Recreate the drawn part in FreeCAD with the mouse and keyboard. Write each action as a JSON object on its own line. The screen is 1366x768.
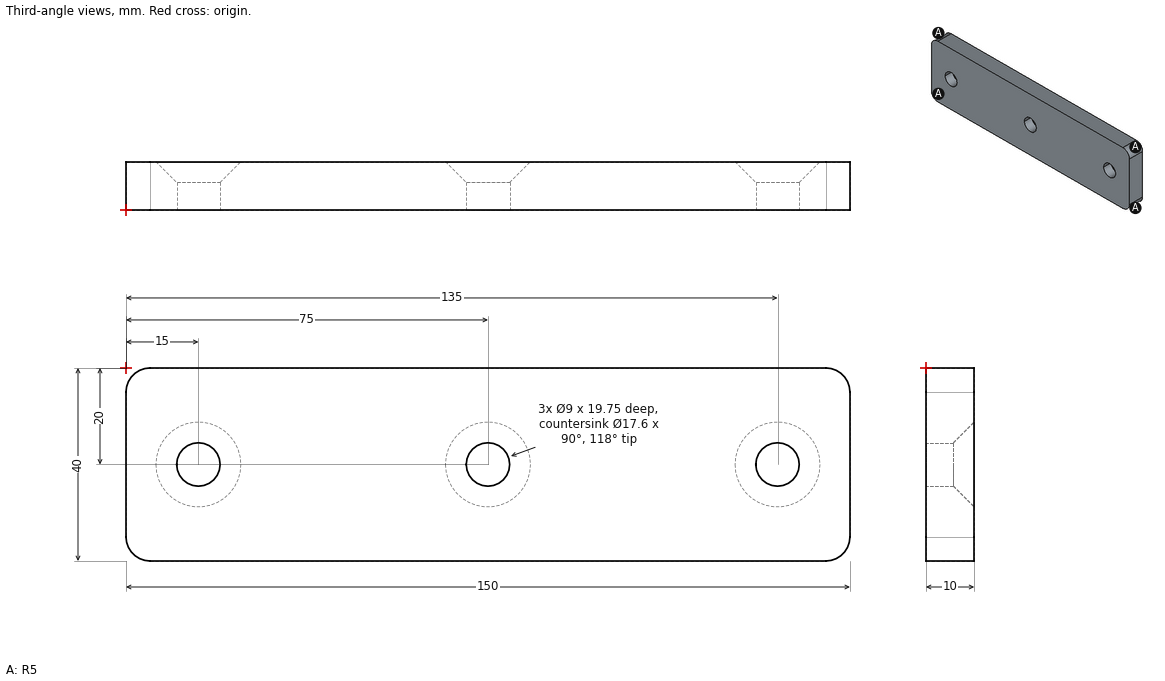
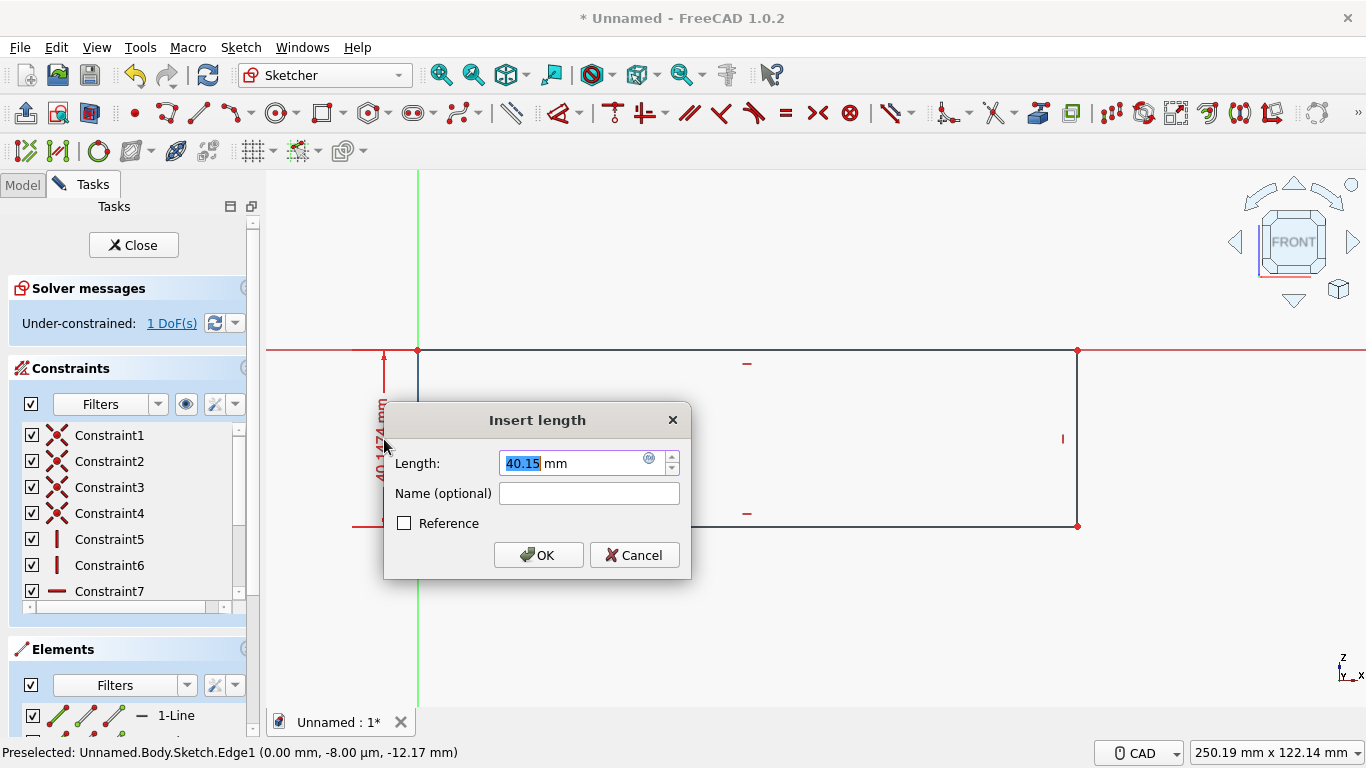
{"action": "type", "text": "40"}
{"action": "key", "text": "Return"}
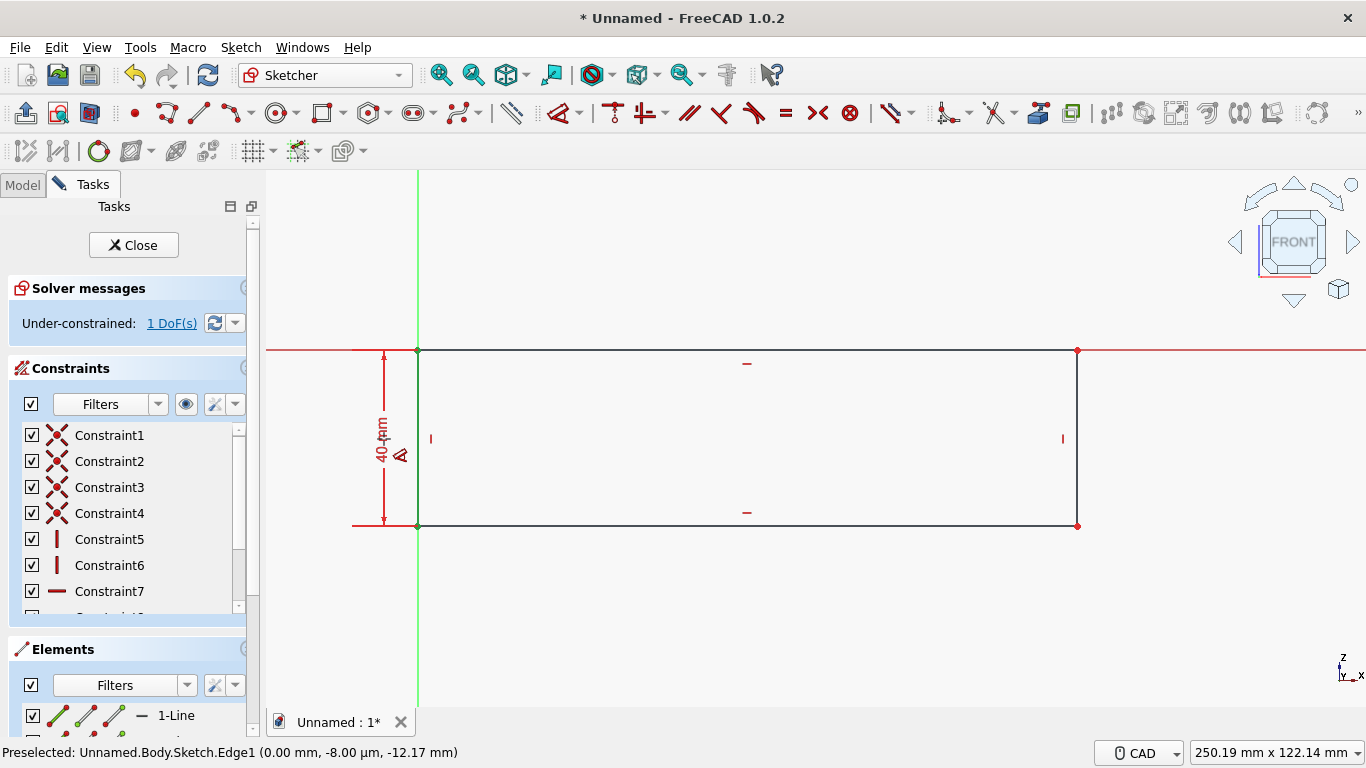
{"action": "left_click", "coordinate": [615, 526]}
{"action": "left_click", "coordinate": [747, 560]}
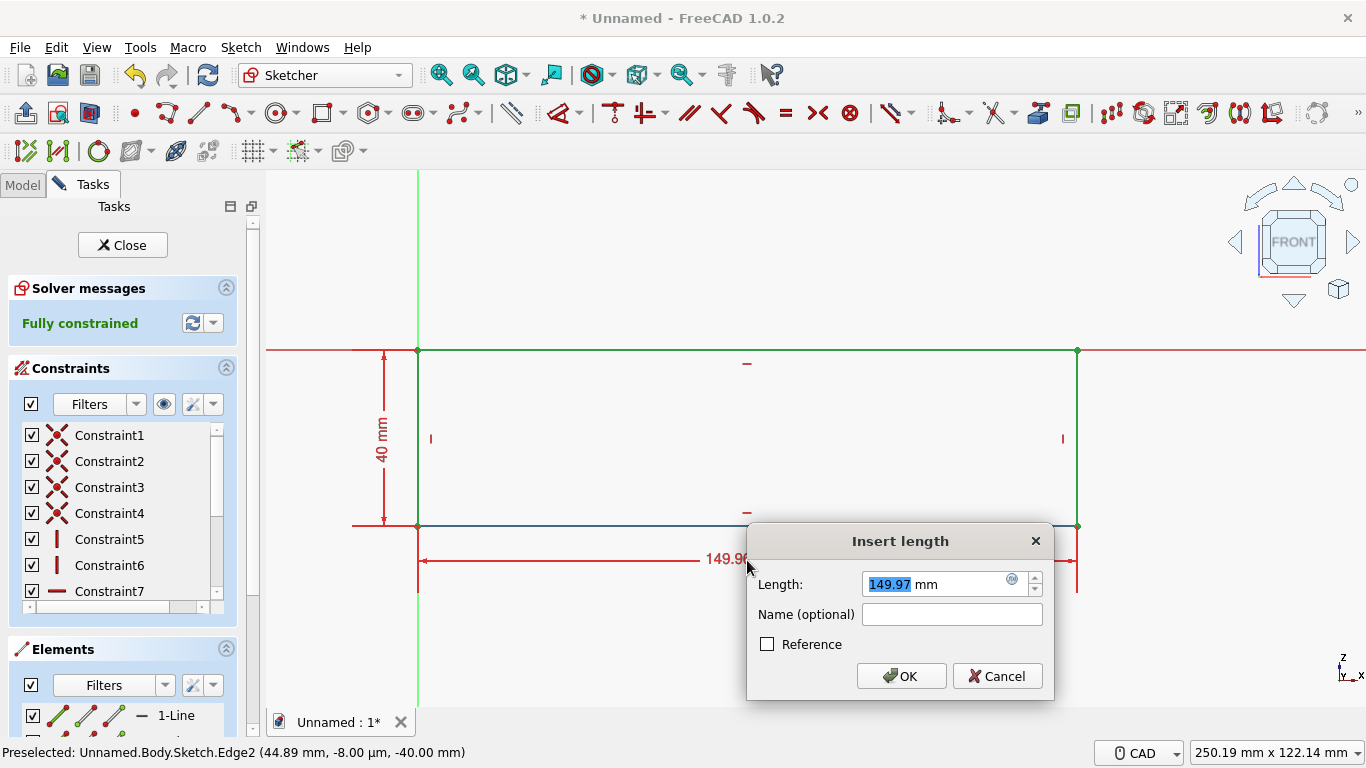
{"action": "type", "text": "150"}
{"action": "key", "text": "Return"}
{"action": "key", "text": "Escape"}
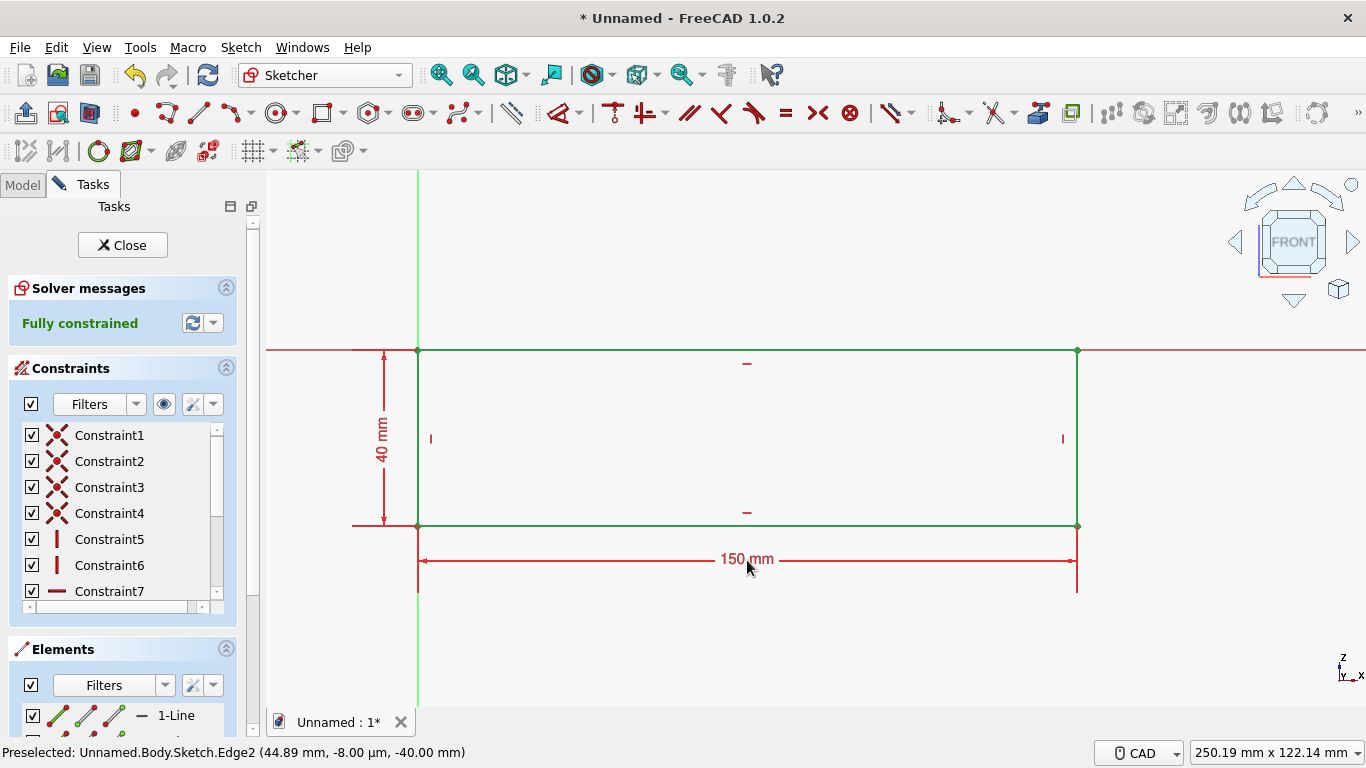
{"action": "left_click", "coordinate": [123, 245]}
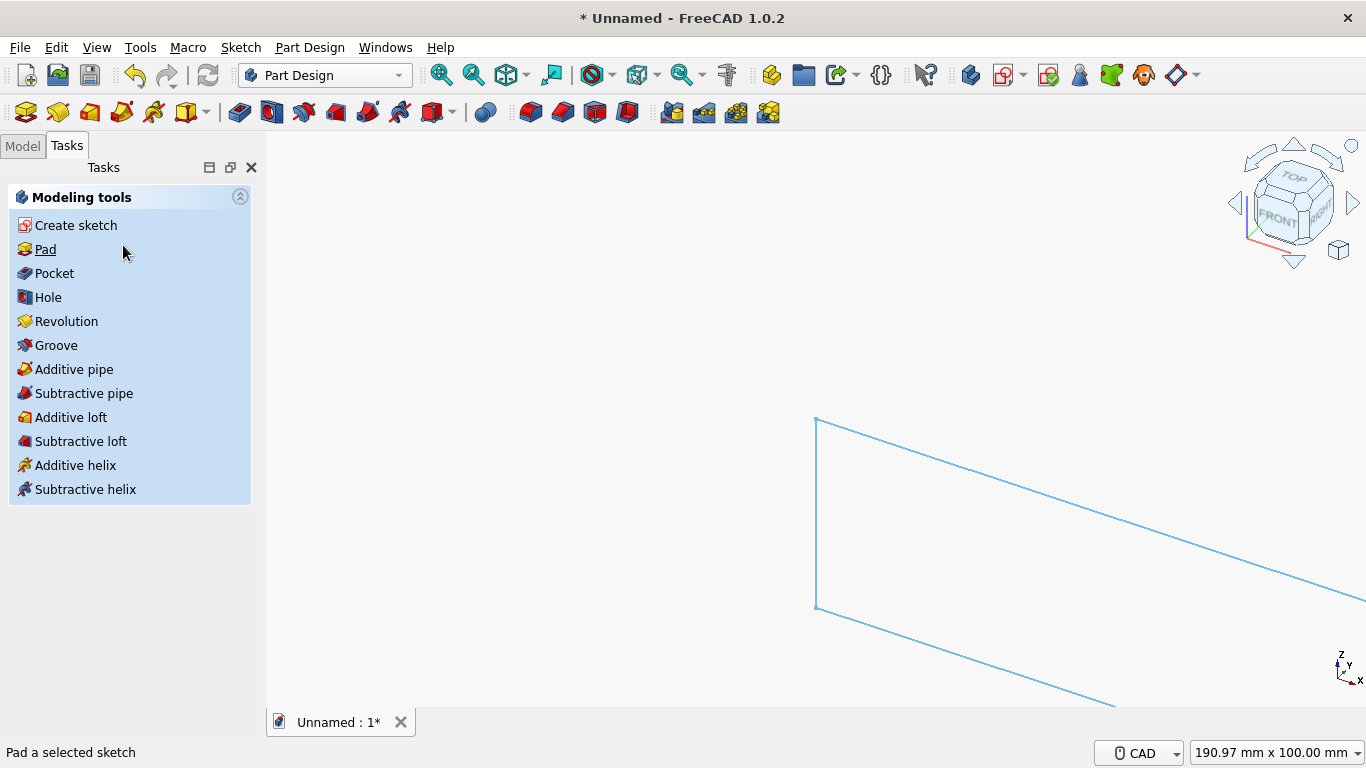
{"action": "left_click", "coordinate": [26, 112]}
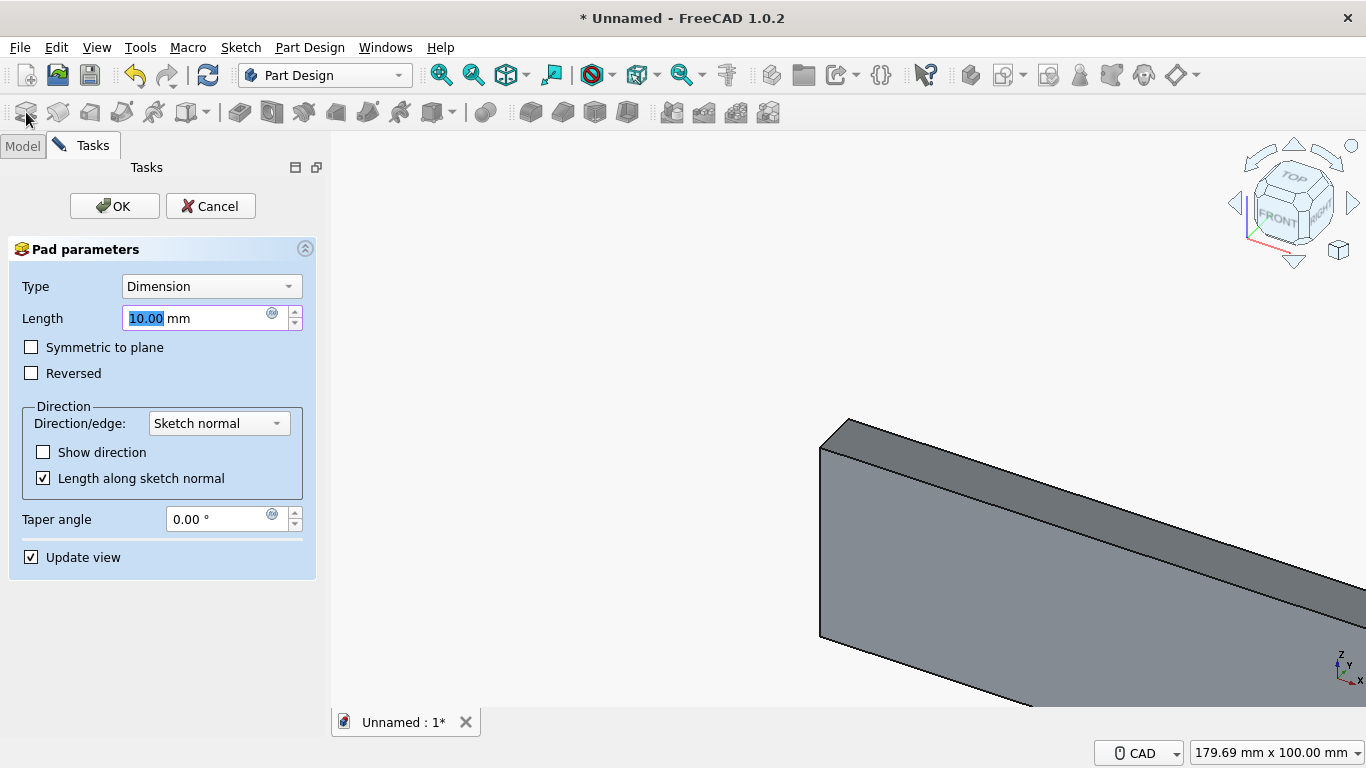
{"action": "type", "text": "10"}
{"action": "key", "text": "Tab"}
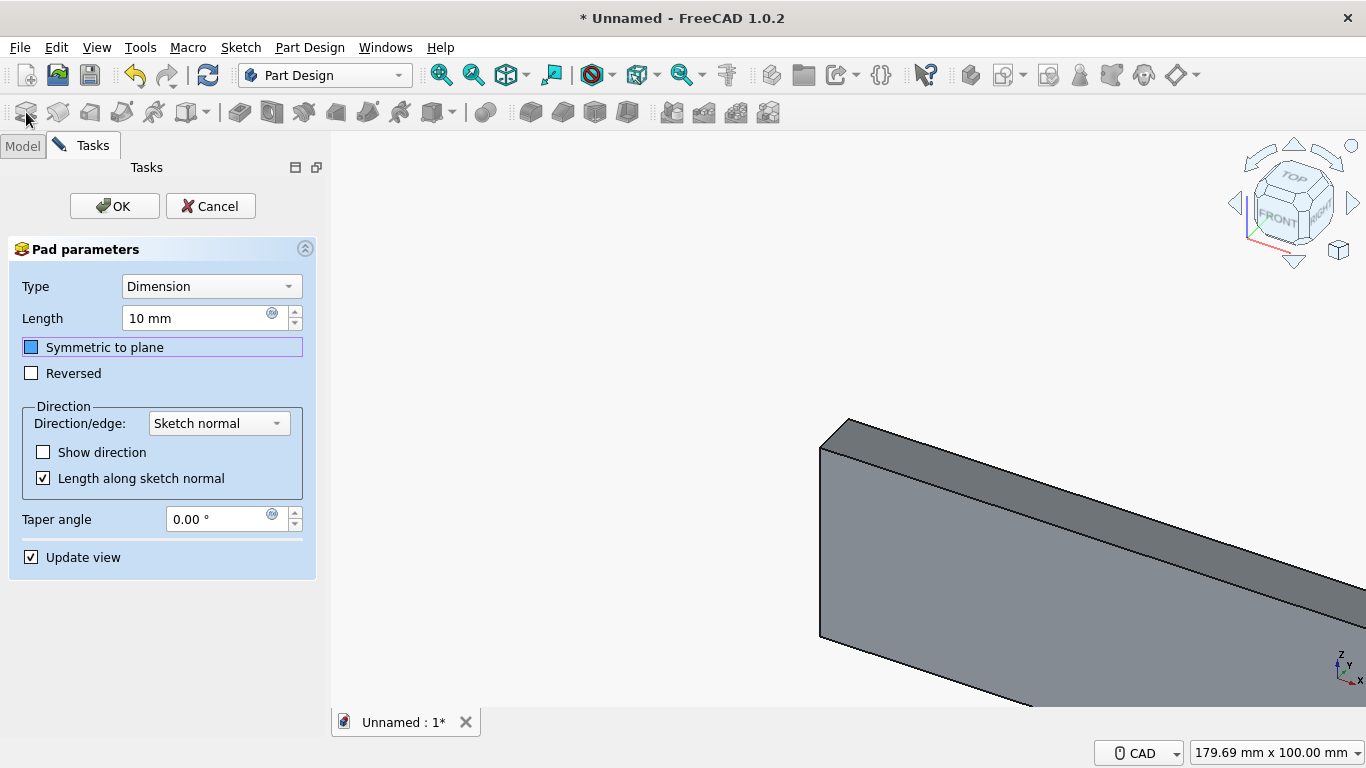
{"action": "left_click", "coordinate": [30, 373]}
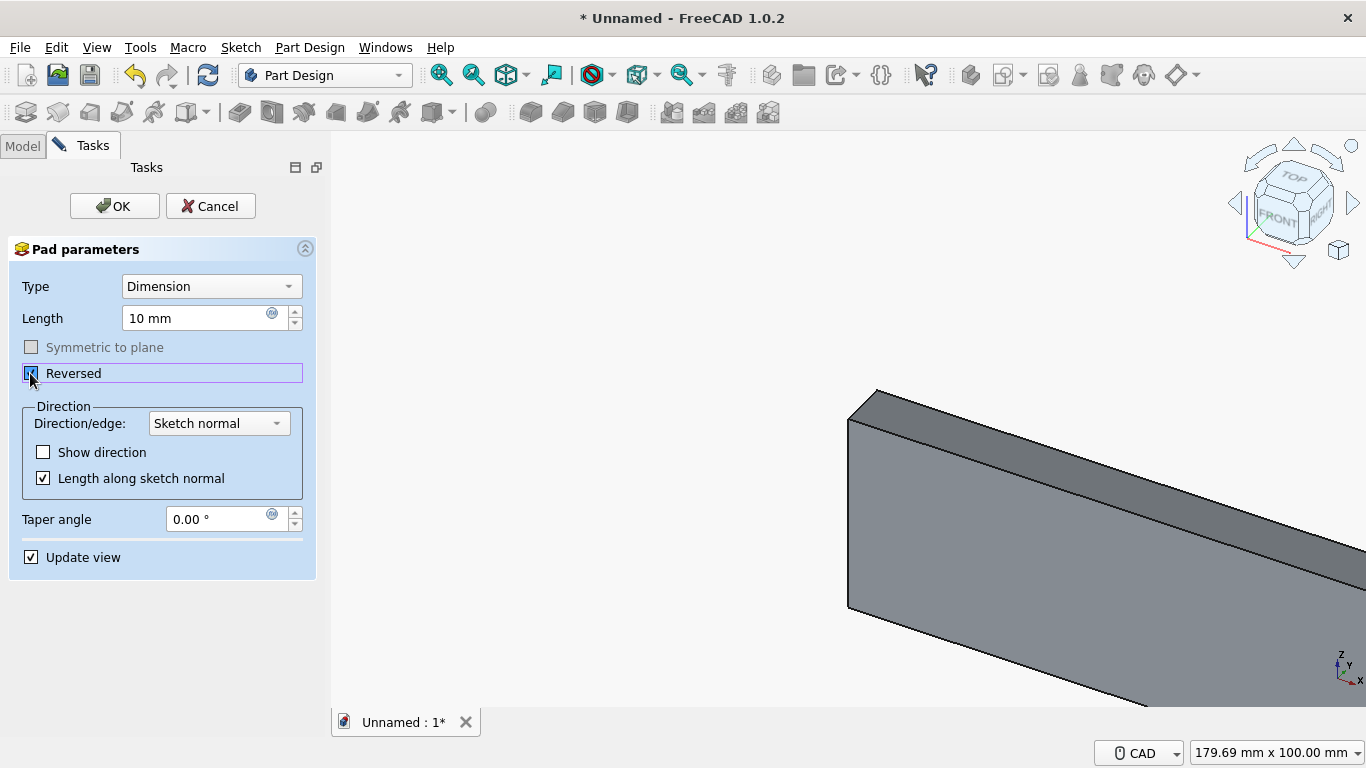
{"action": "left_click", "coordinate": [115, 206]}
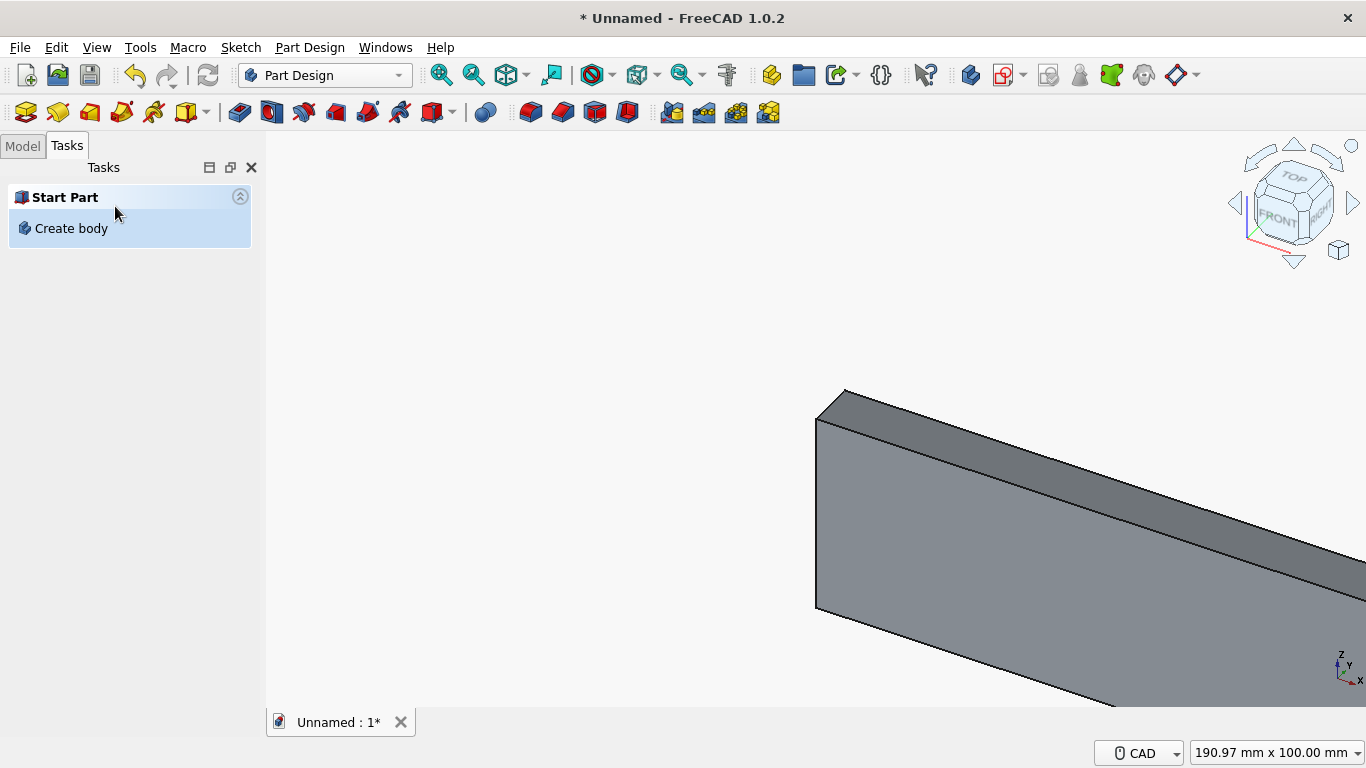
{"action": "left_click", "coordinate": [442, 76]}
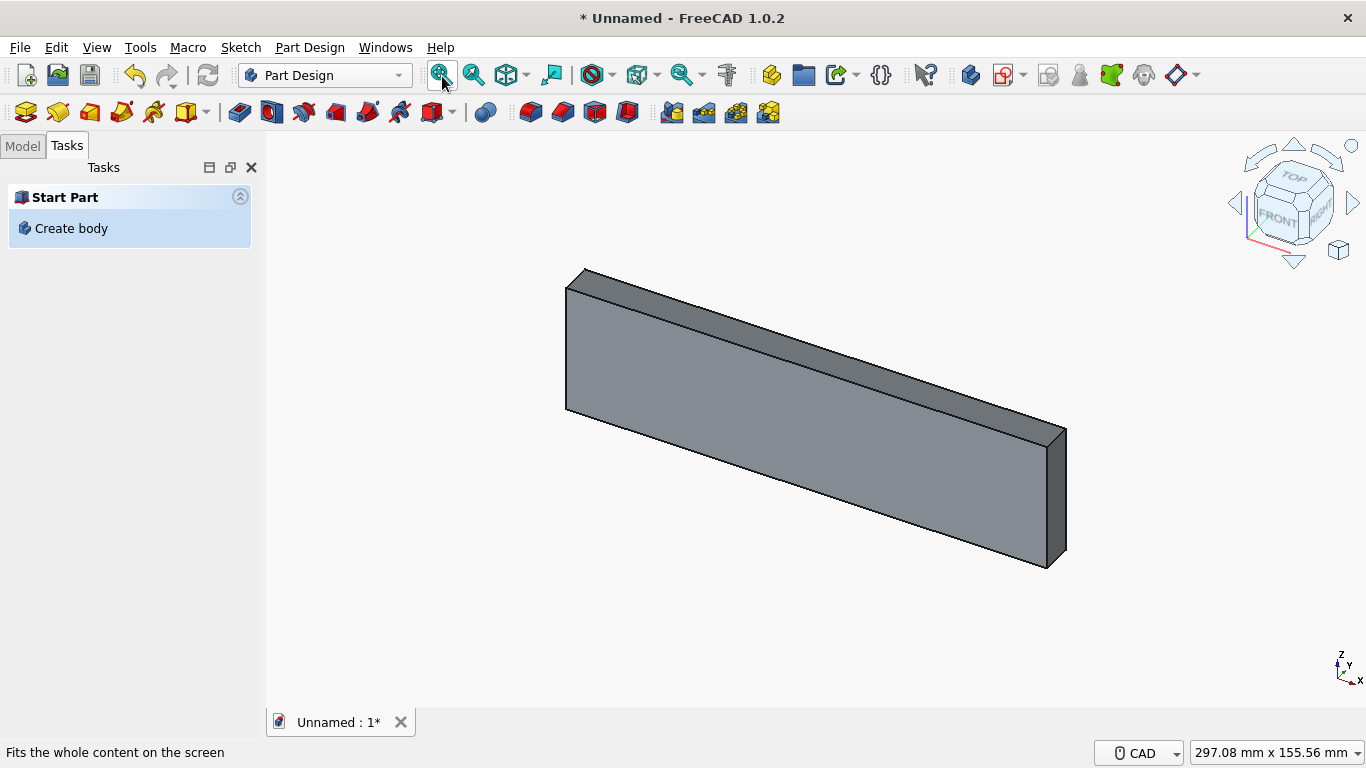
{"action": "left_click", "coordinate": [1056, 437]}